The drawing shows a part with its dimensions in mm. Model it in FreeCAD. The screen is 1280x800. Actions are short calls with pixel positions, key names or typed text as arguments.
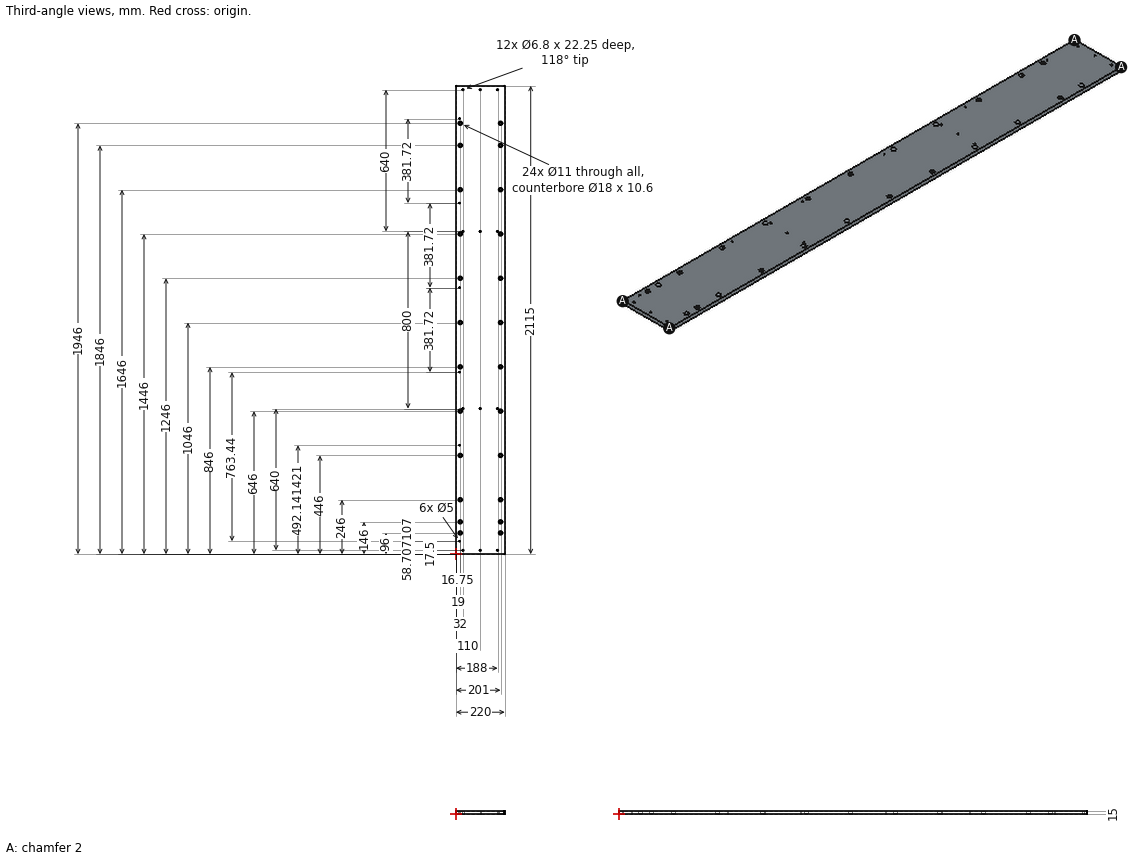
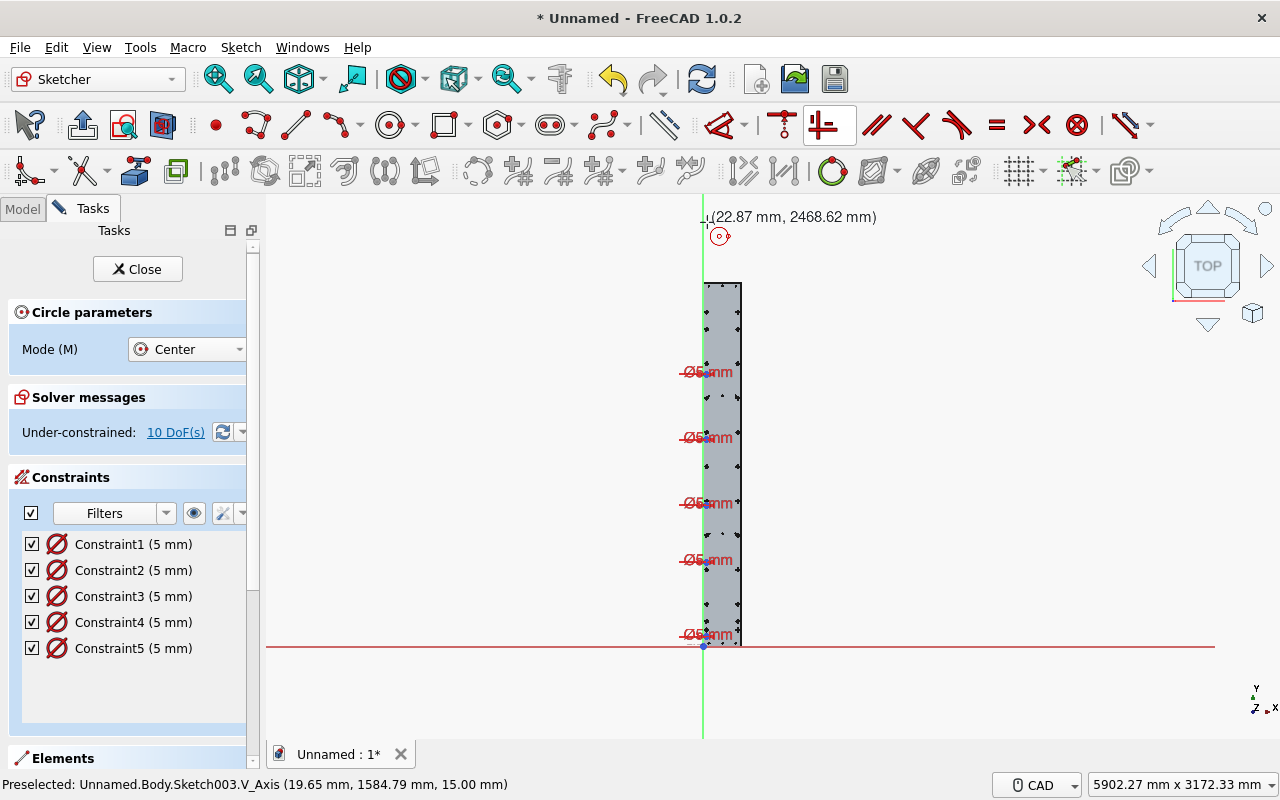
scroll(706, 309, up, 9)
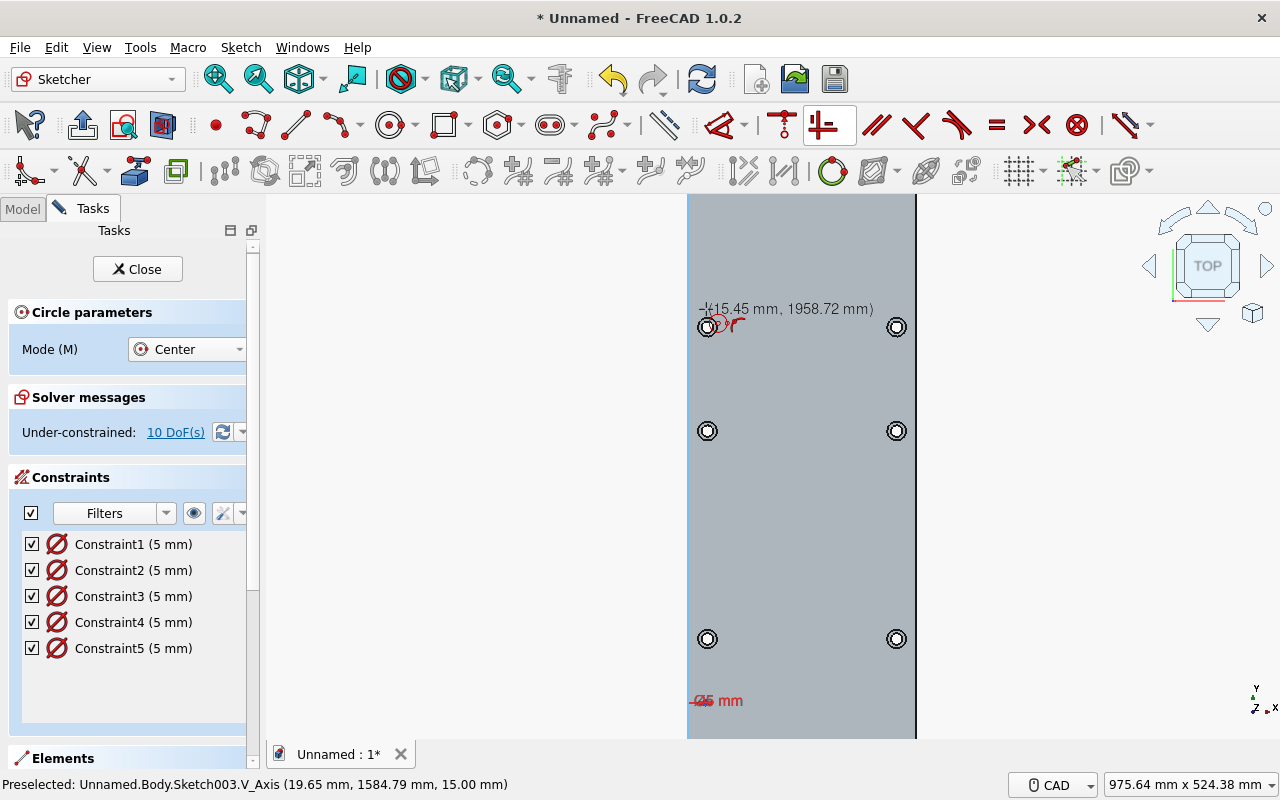
click(705, 305)
move(707, 303)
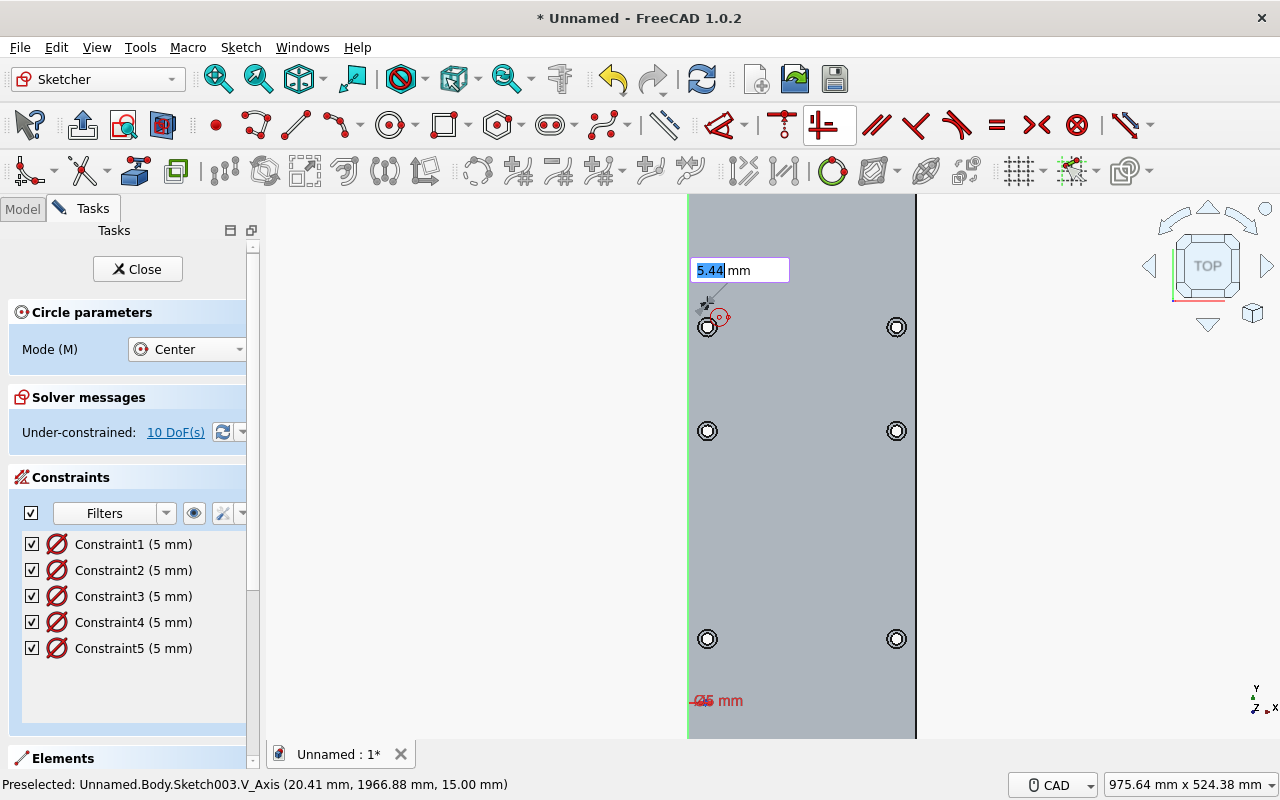
text(5)
key(Return)
key(Escape)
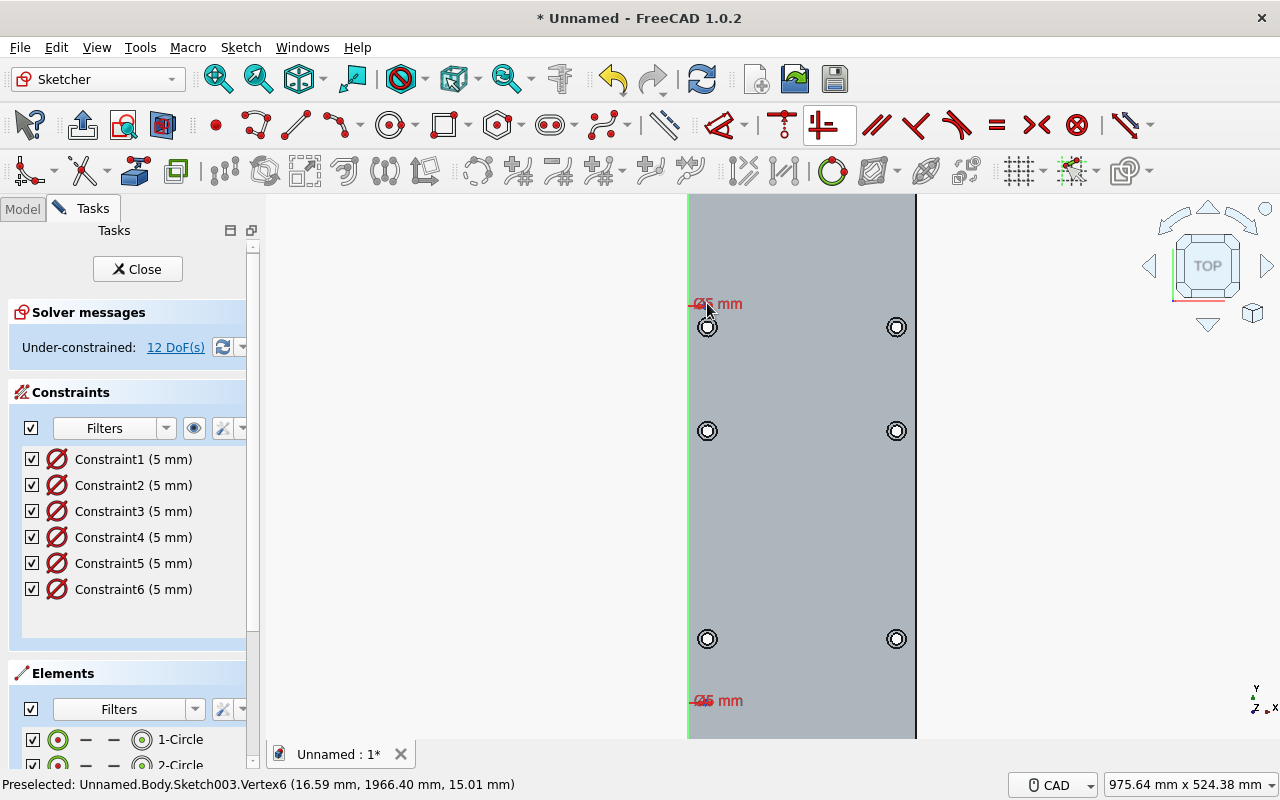
scroll(706, 296, down, 9)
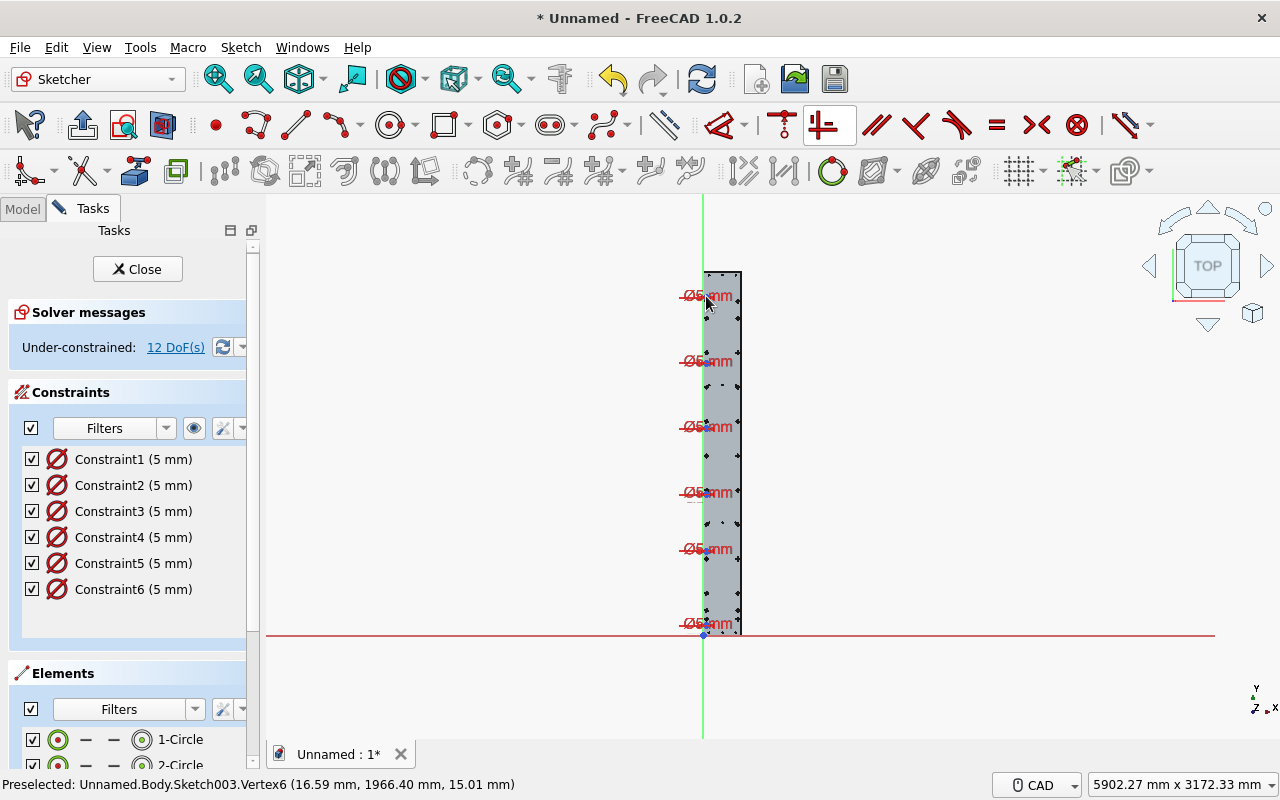
click(706, 626)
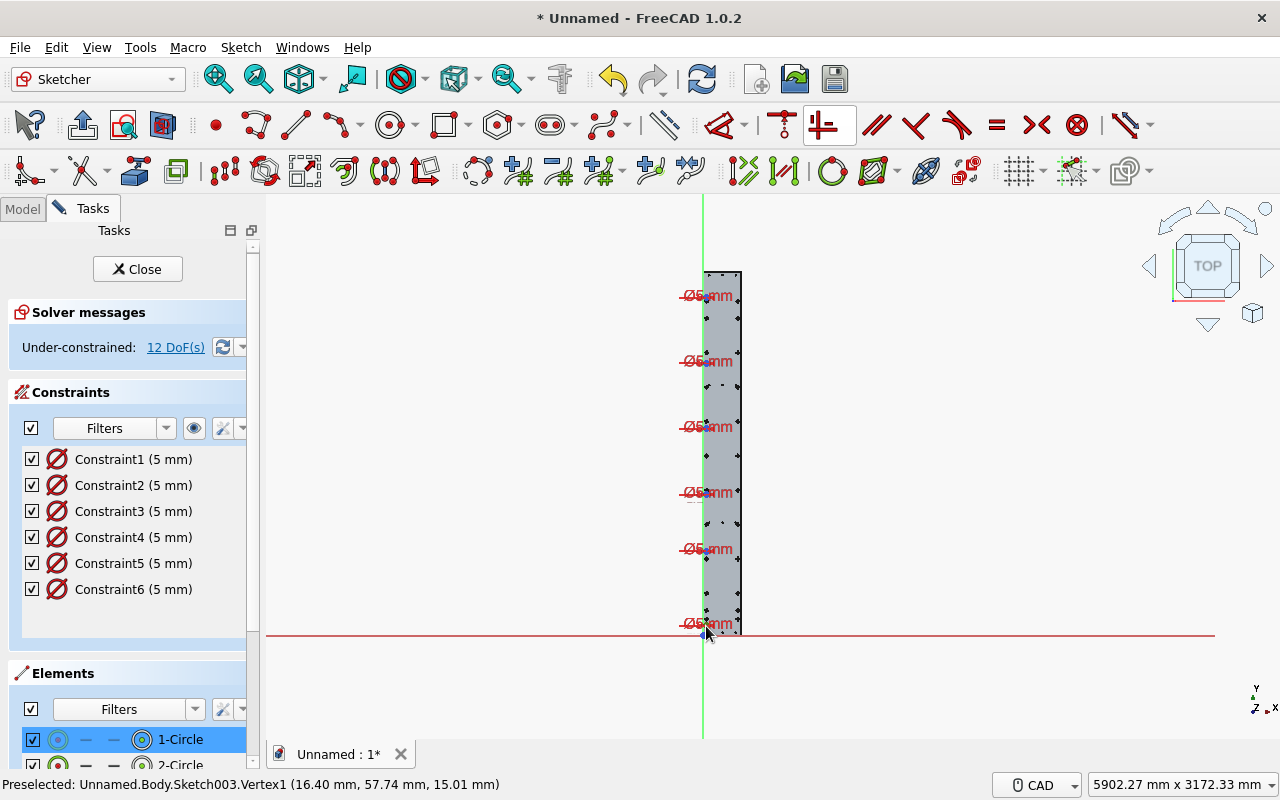
click(706, 551)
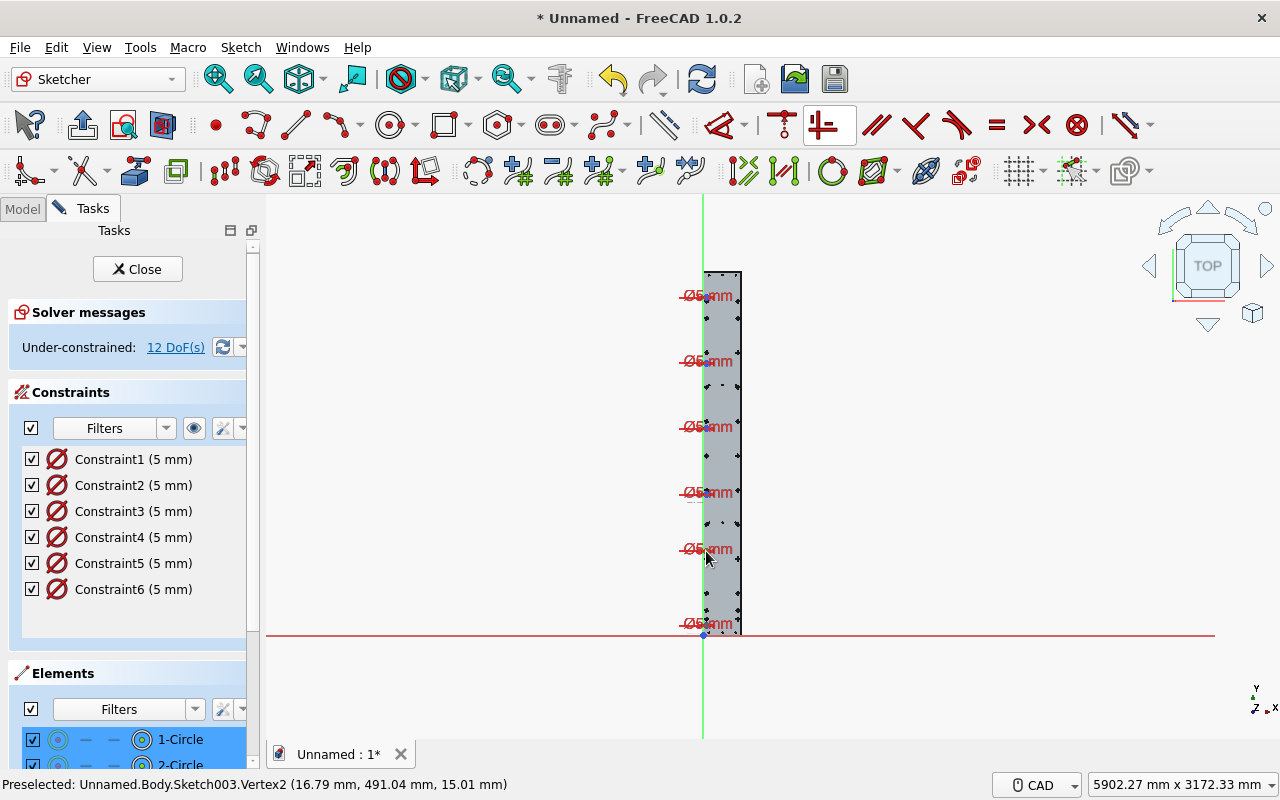
key(v)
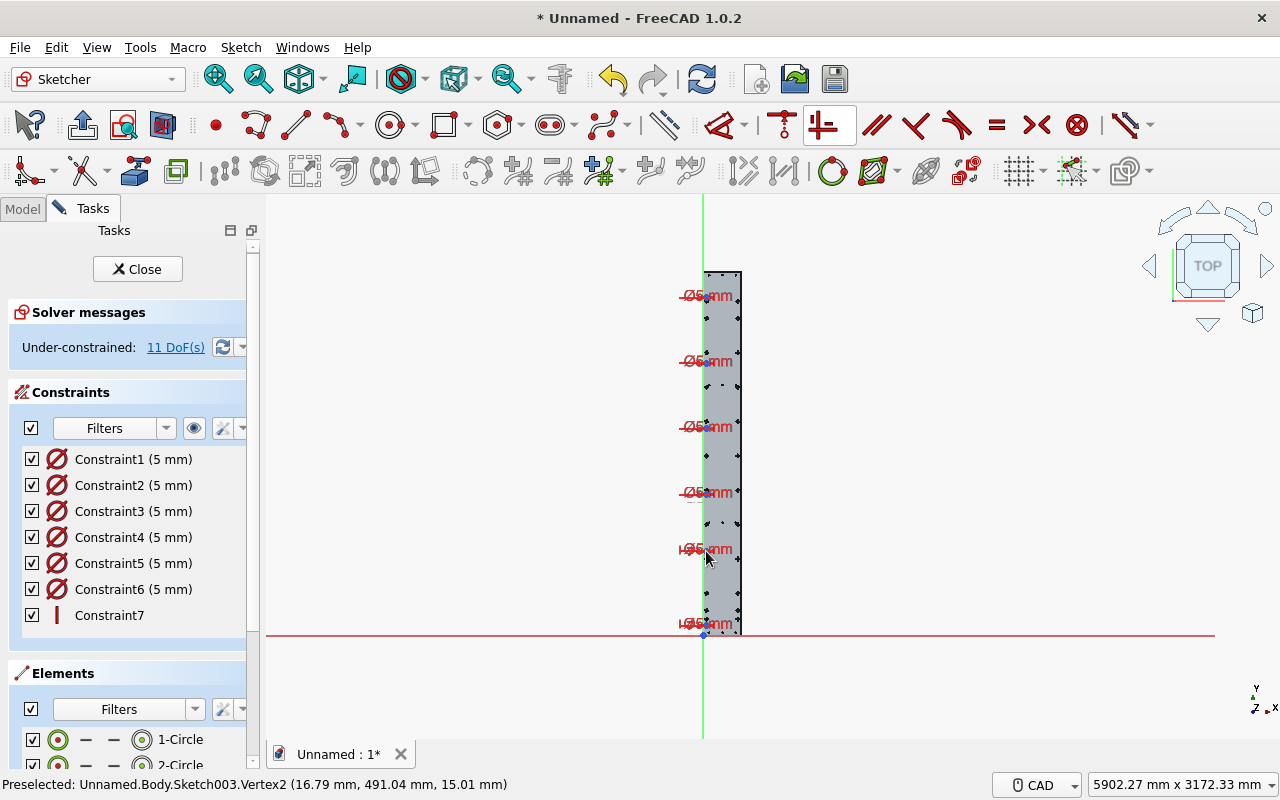
click(706, 551)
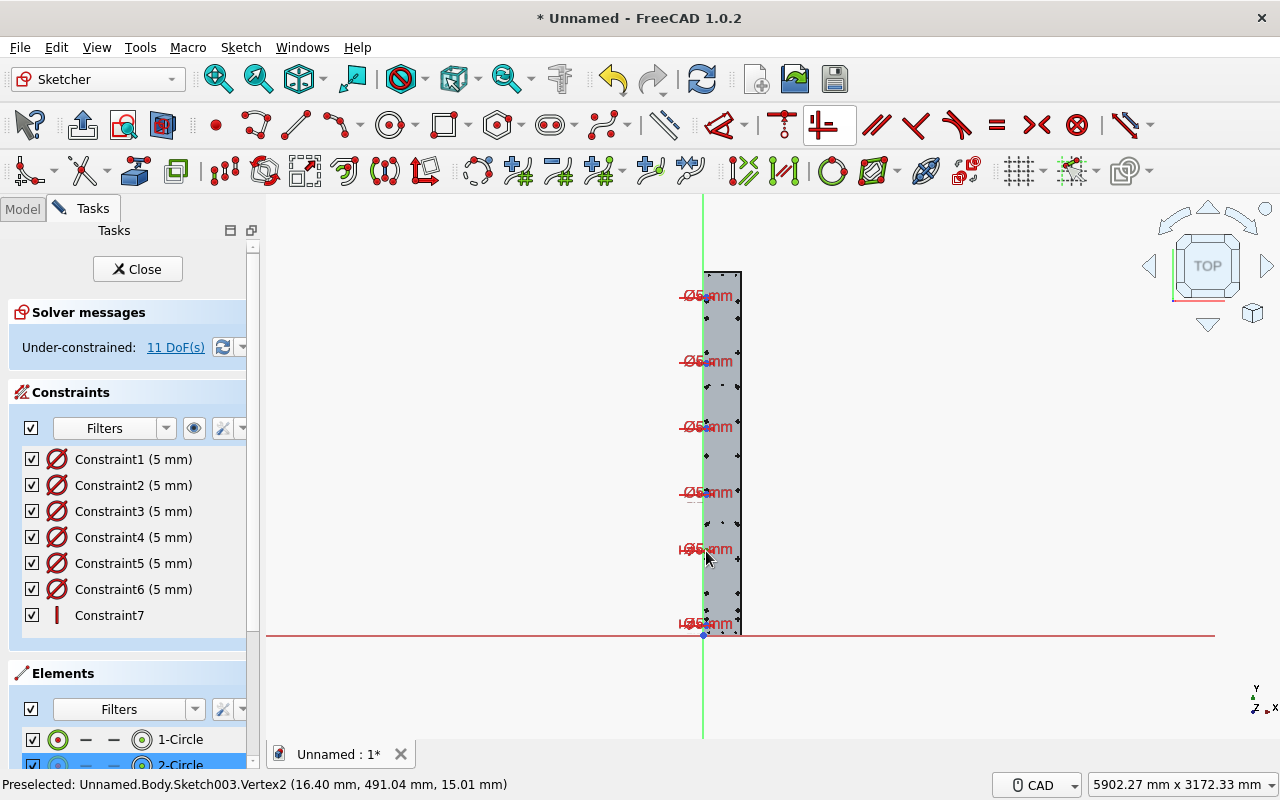
click(706, 495)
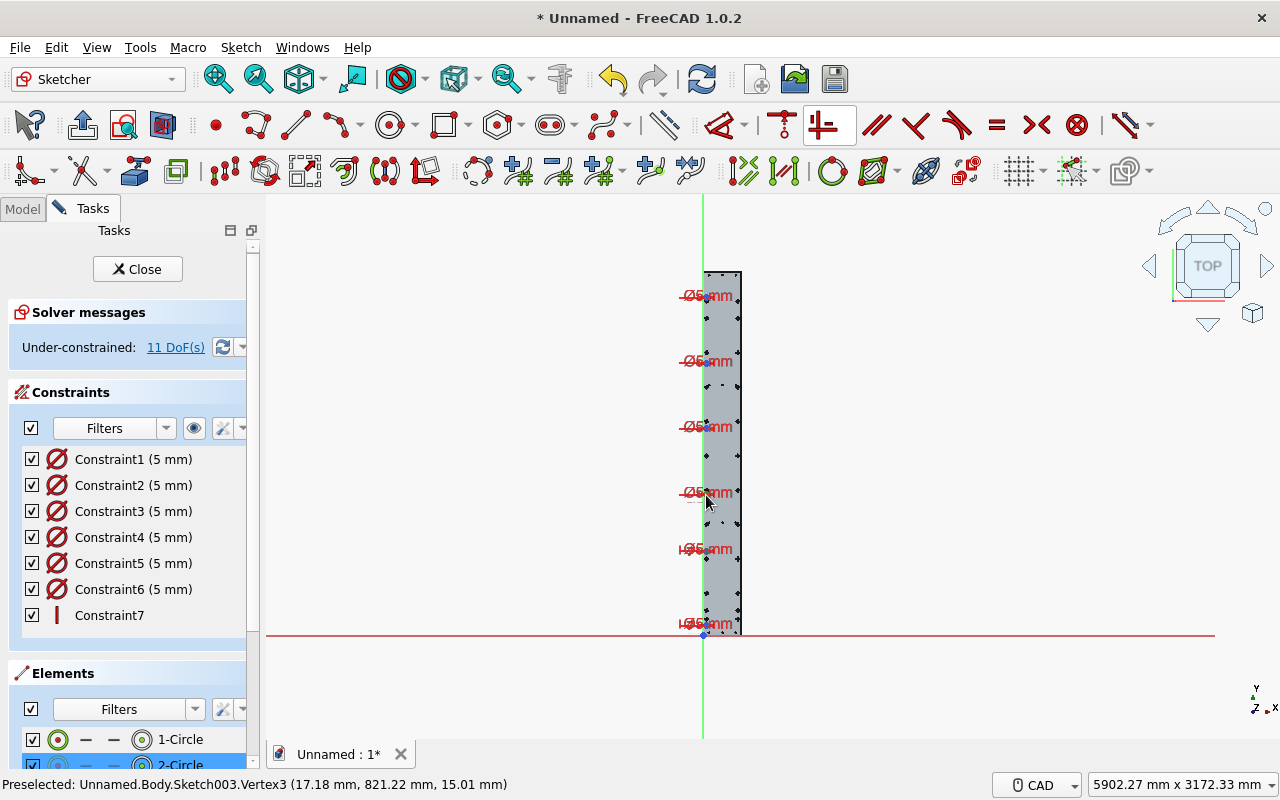
click(850, 126)